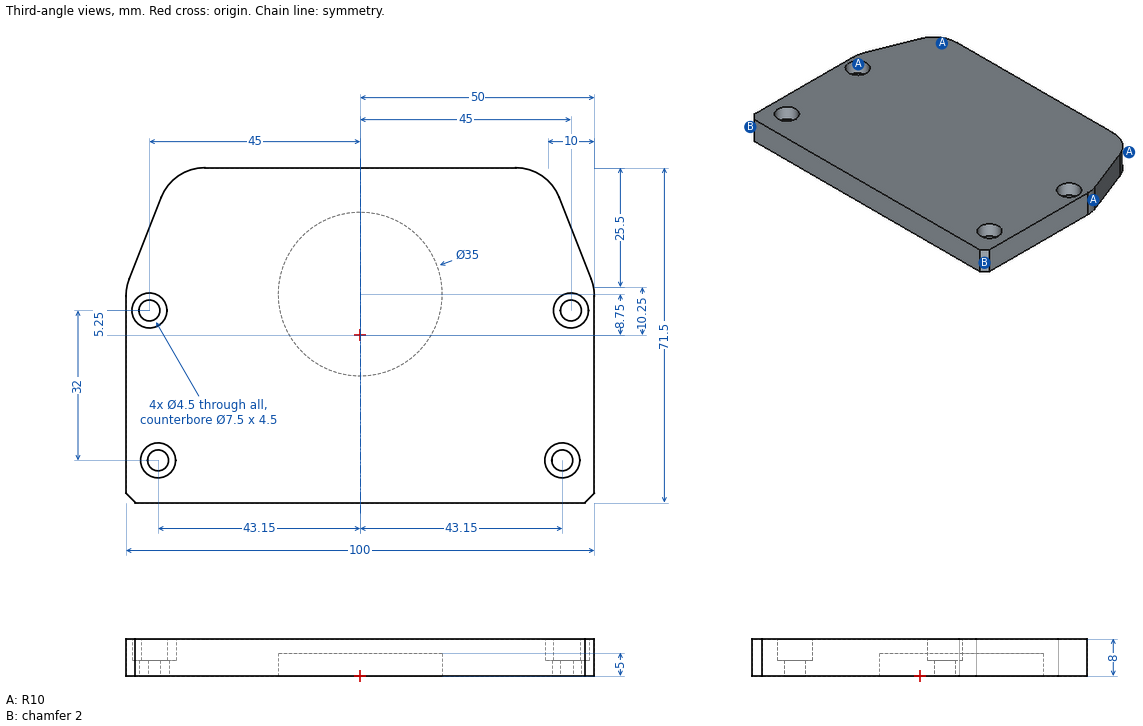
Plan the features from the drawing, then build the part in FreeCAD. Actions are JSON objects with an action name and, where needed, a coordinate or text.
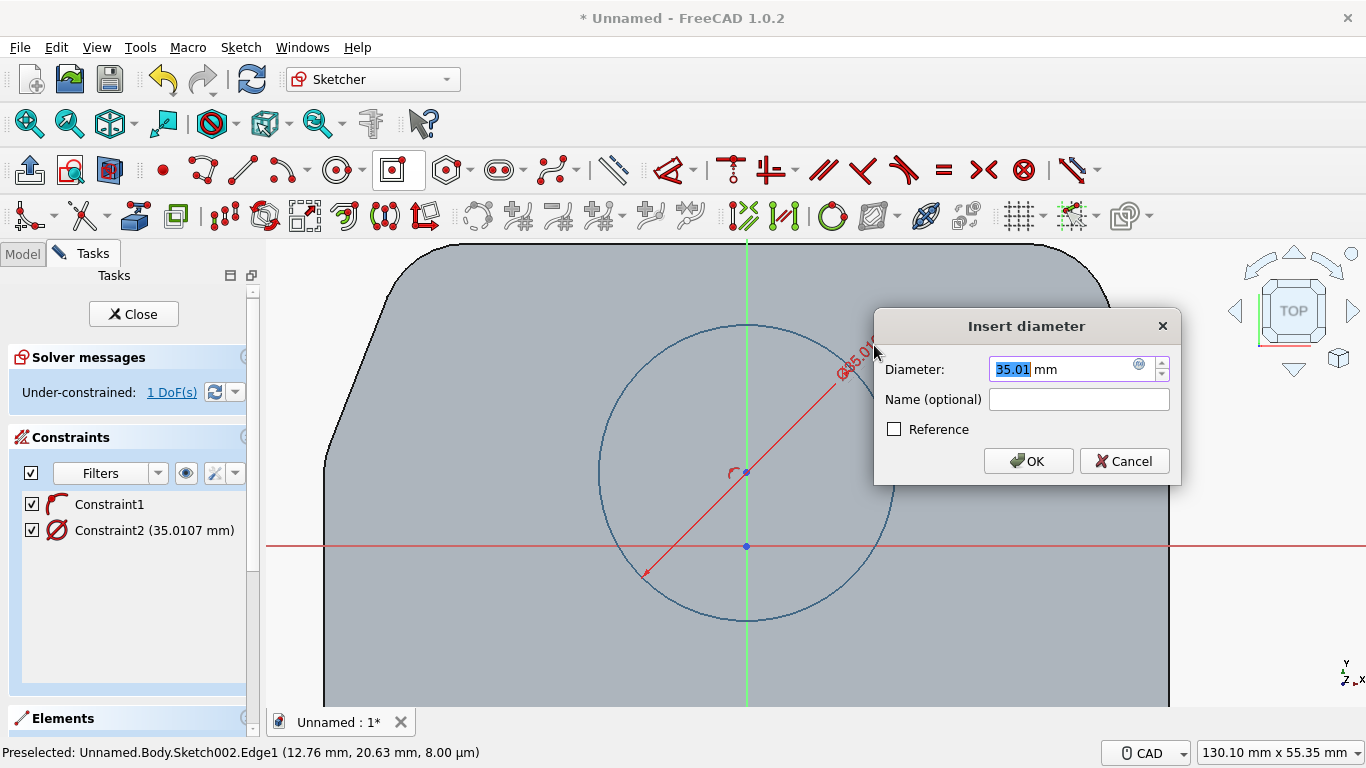
{"action": "type", "text": "35"}
{"action": "key", "text": "Return"}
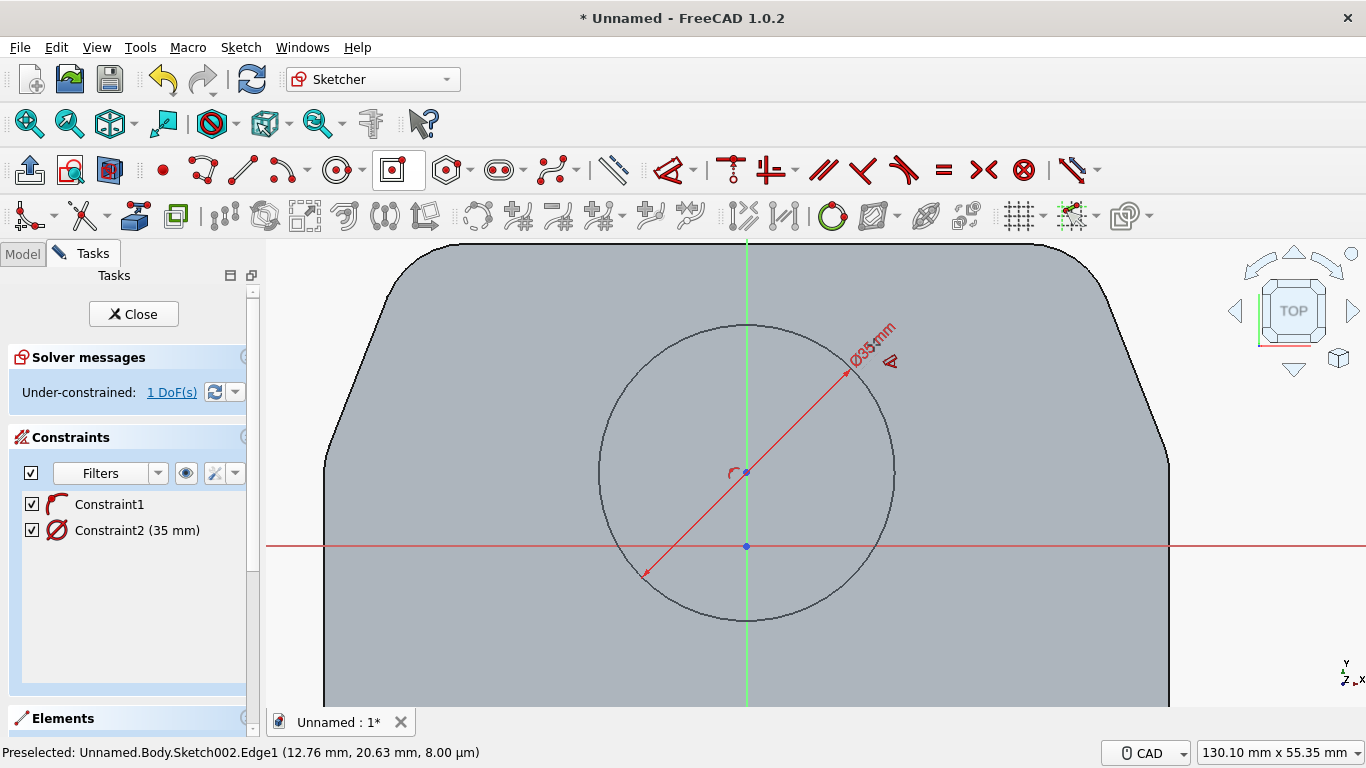
{"action": "left_click", "coordinate": [747, 473]}
{"action": "left_click", "coordinate": [781, 510]}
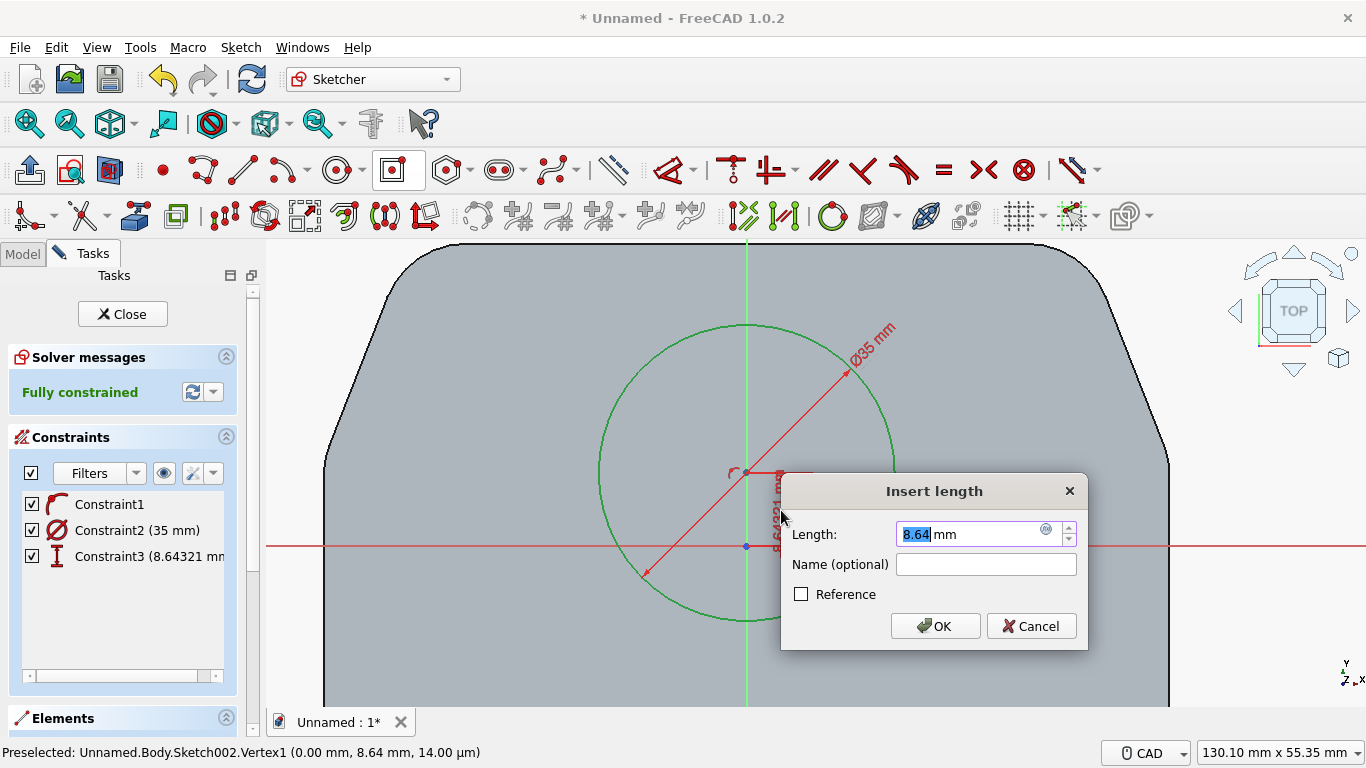
{"action": "type", "text": "8.75"}
{"action": "key", "text": "Return"}
{"action": "key", "text": "Escape"}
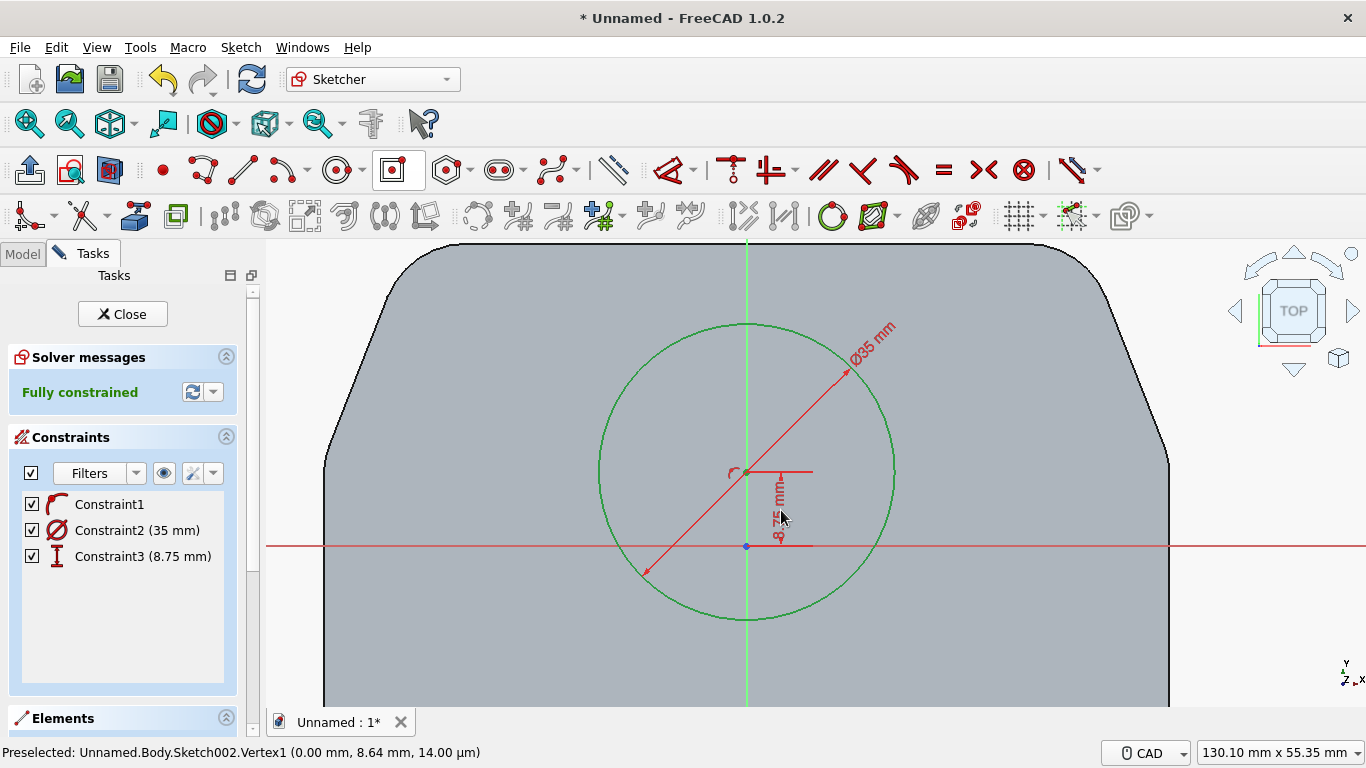
{"action": "left_click", "coordinate": [123, 314]}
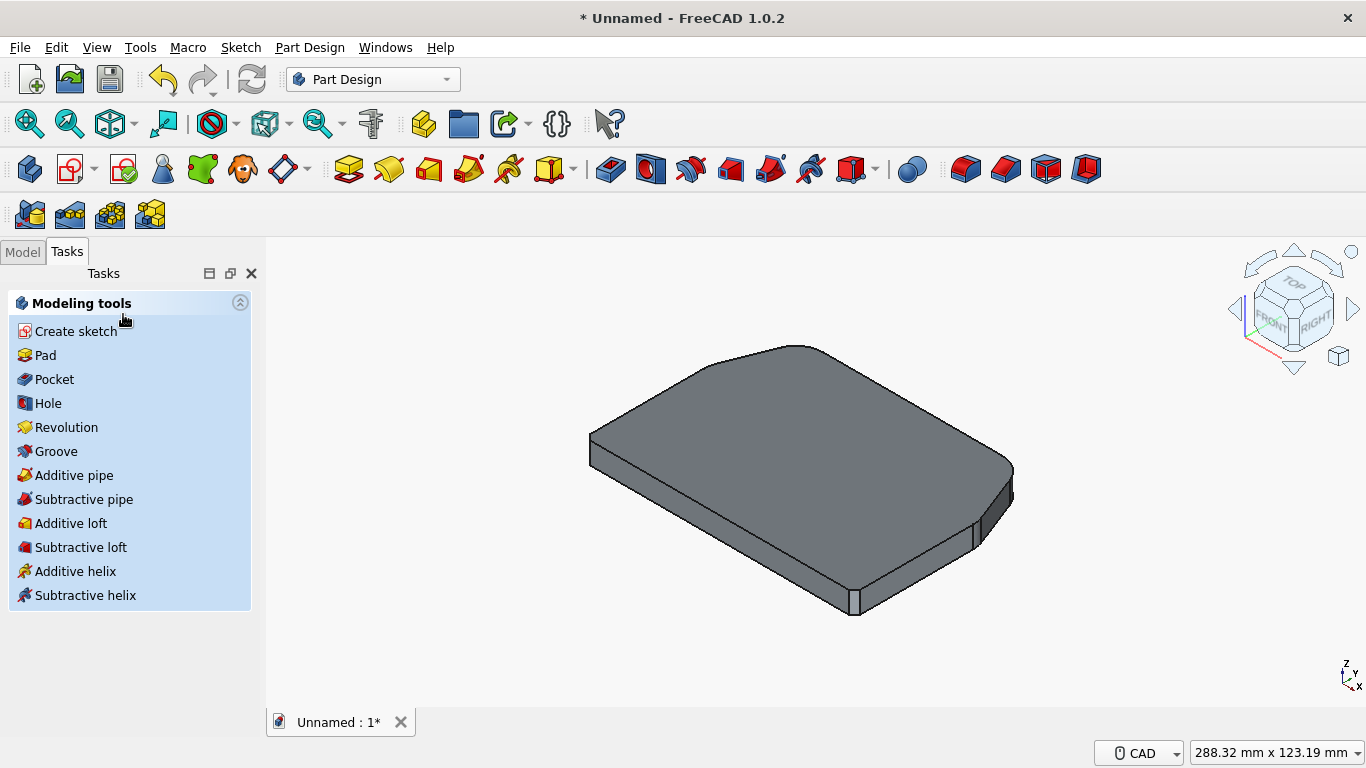
{"action": "left_click", "coordinate": [612, 170]}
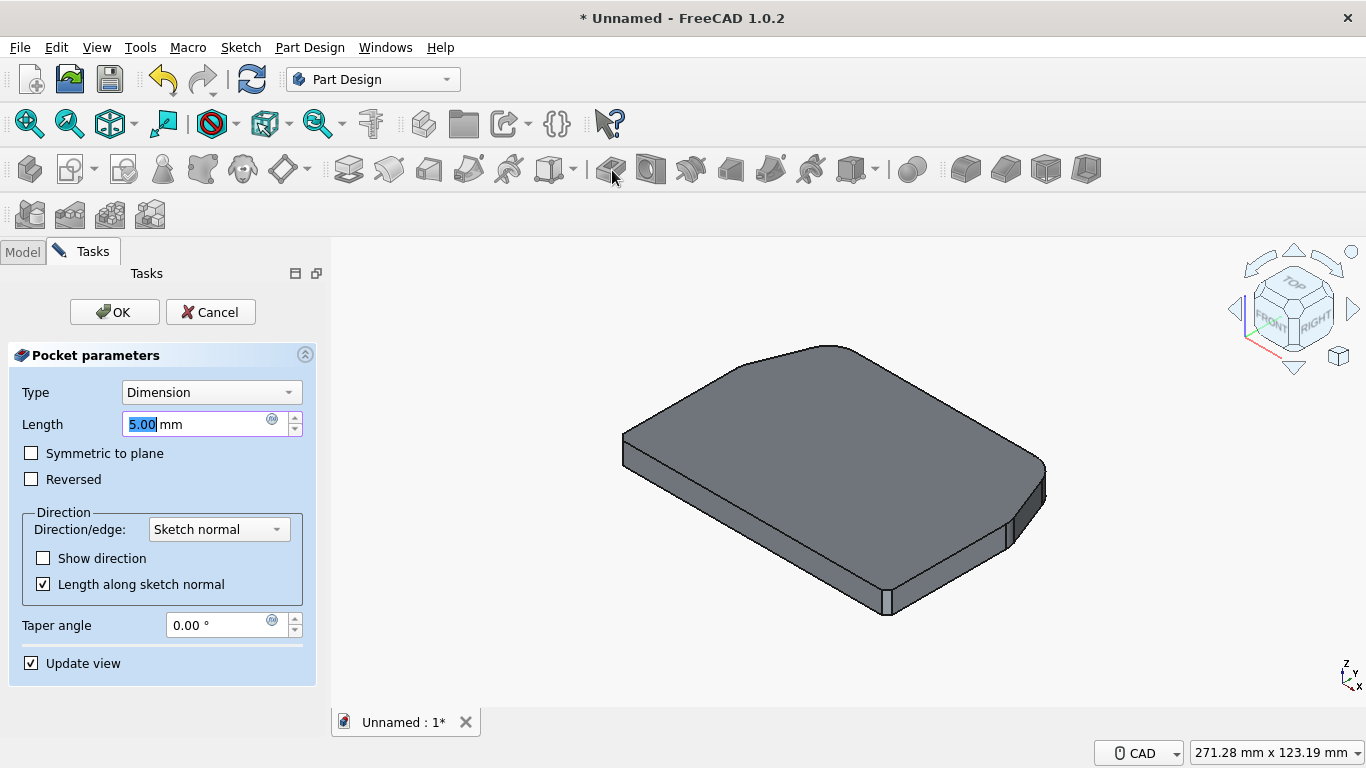
{"action": "type", "text": "5"}
{"action": "key", "text": "Tab"}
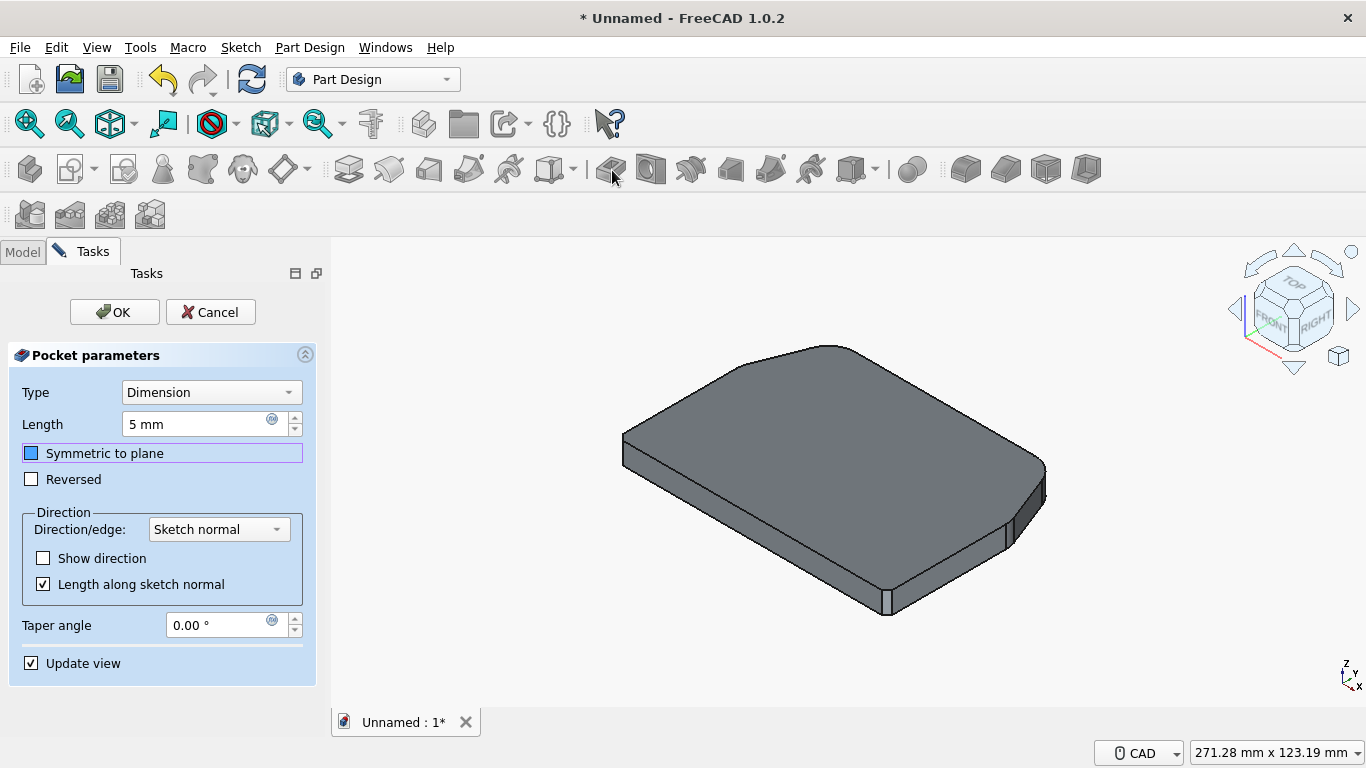
{"action": "left_click", "coordinate": [30, 479]}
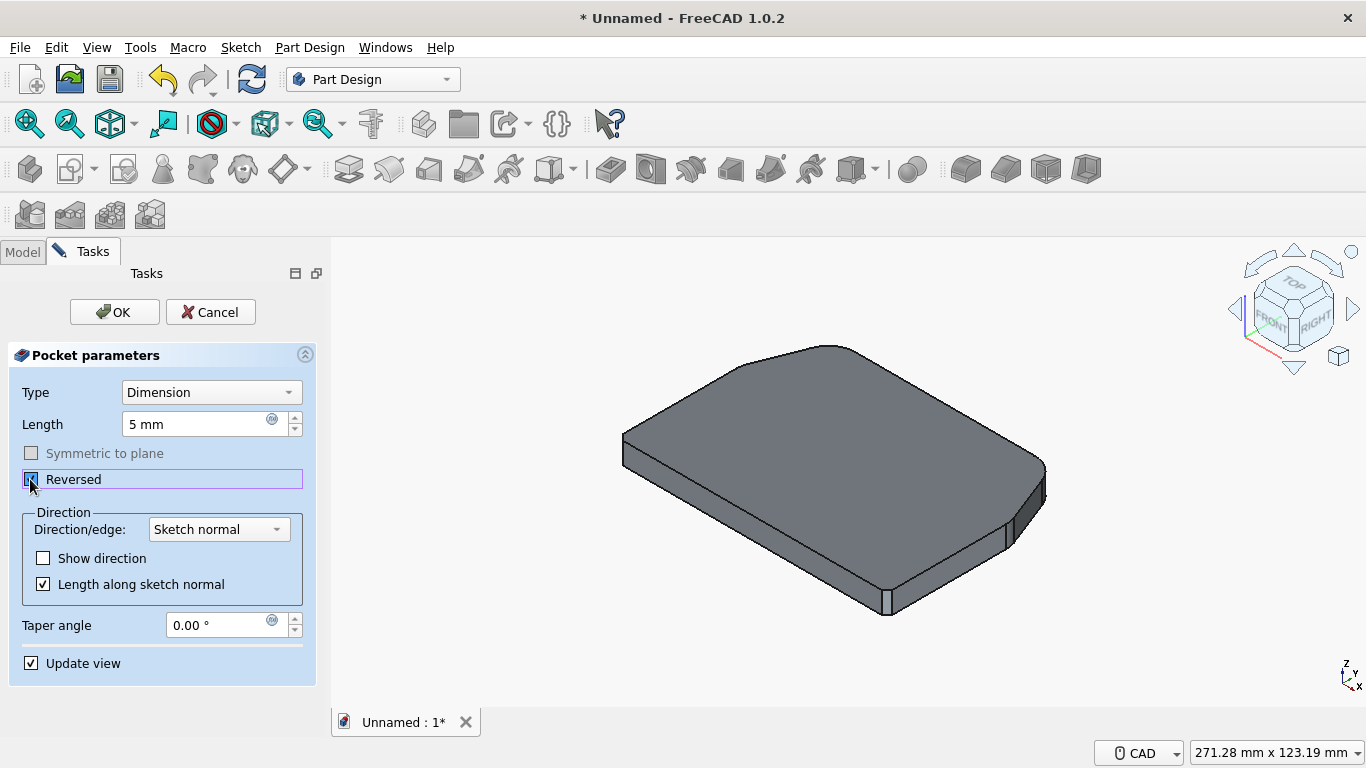
{"action": "left_click", "coordinate": [115, 312]}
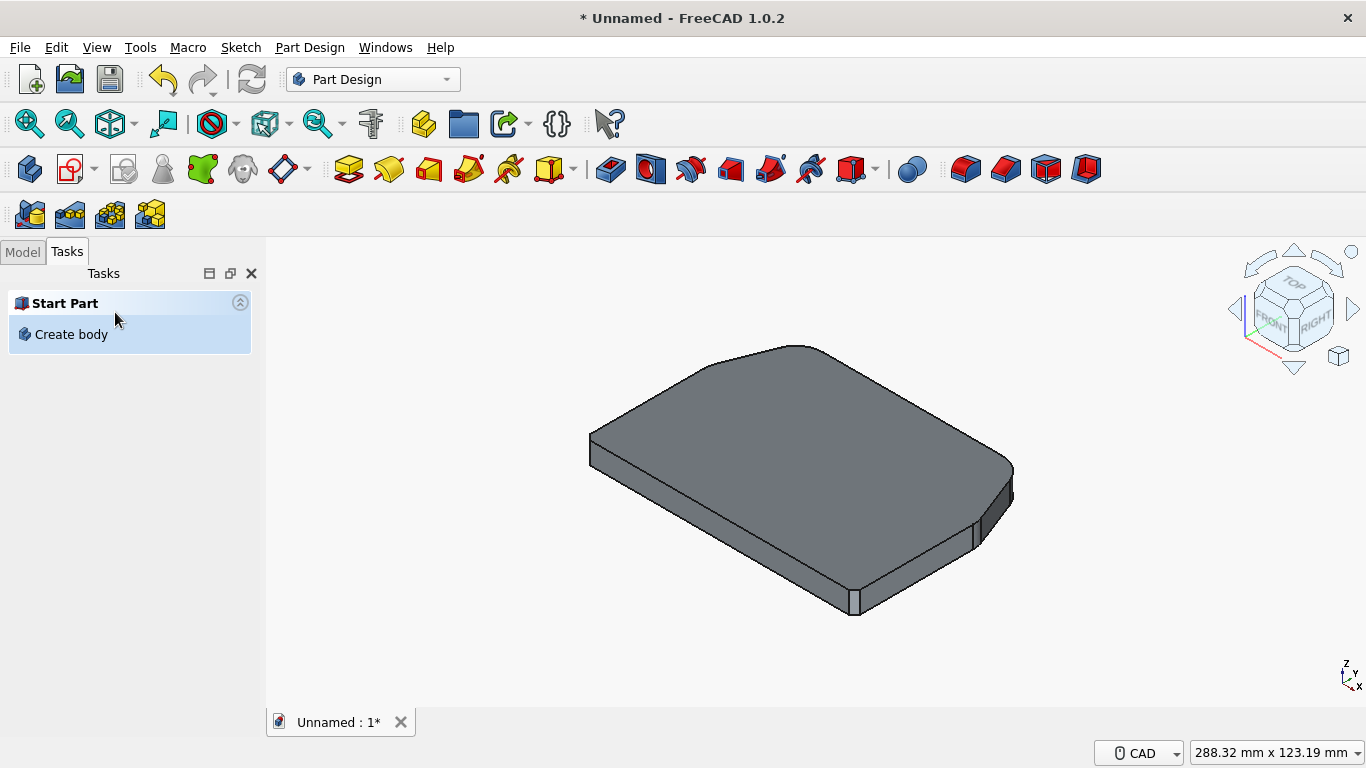
{"action": "left_click", "coordinate": [816, 459]}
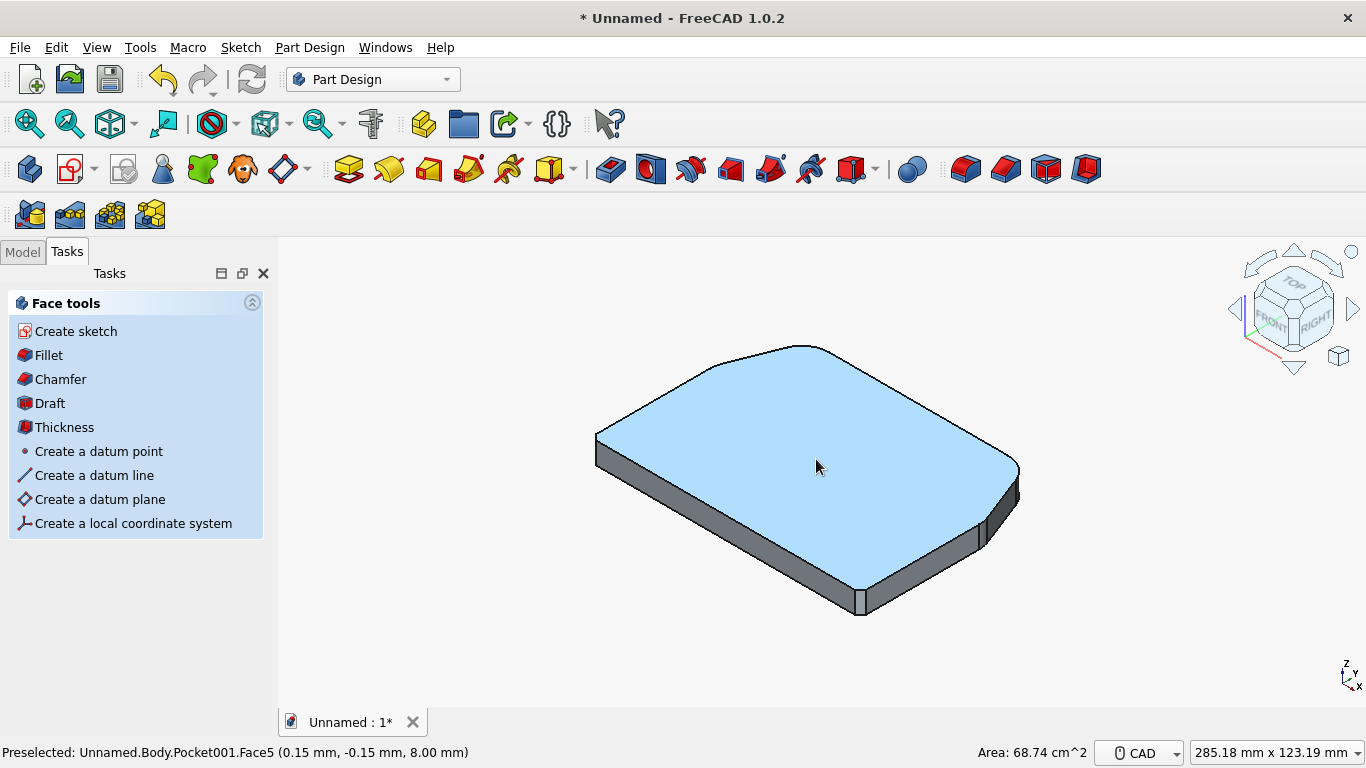
{"action": "left_click", "coordinate": [70, 170]}